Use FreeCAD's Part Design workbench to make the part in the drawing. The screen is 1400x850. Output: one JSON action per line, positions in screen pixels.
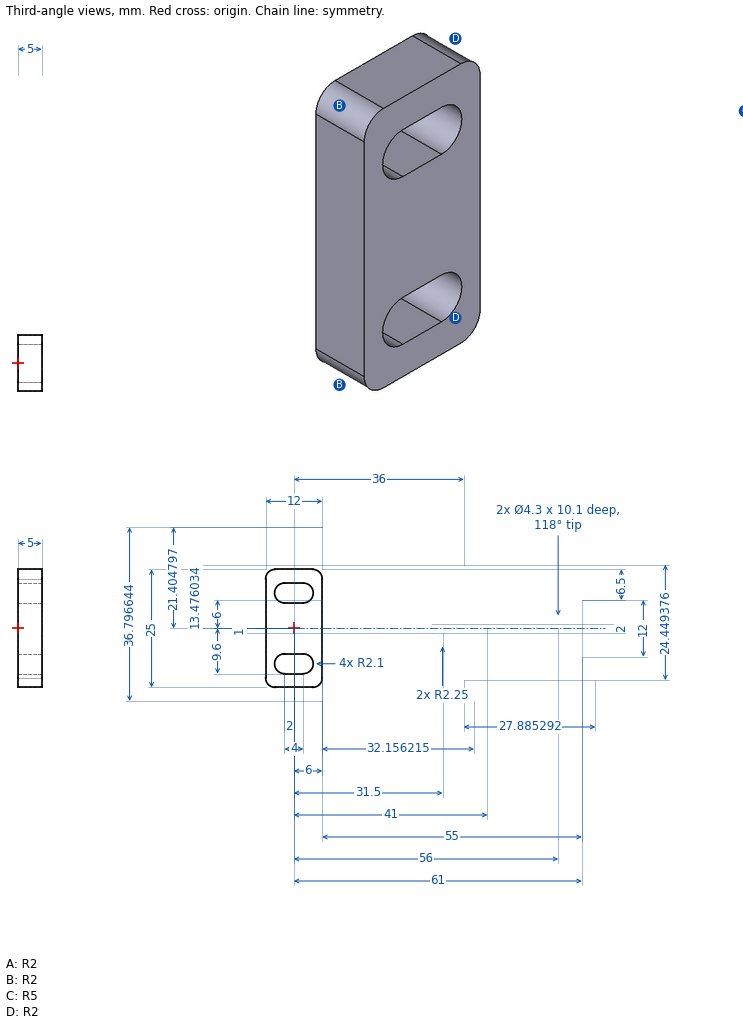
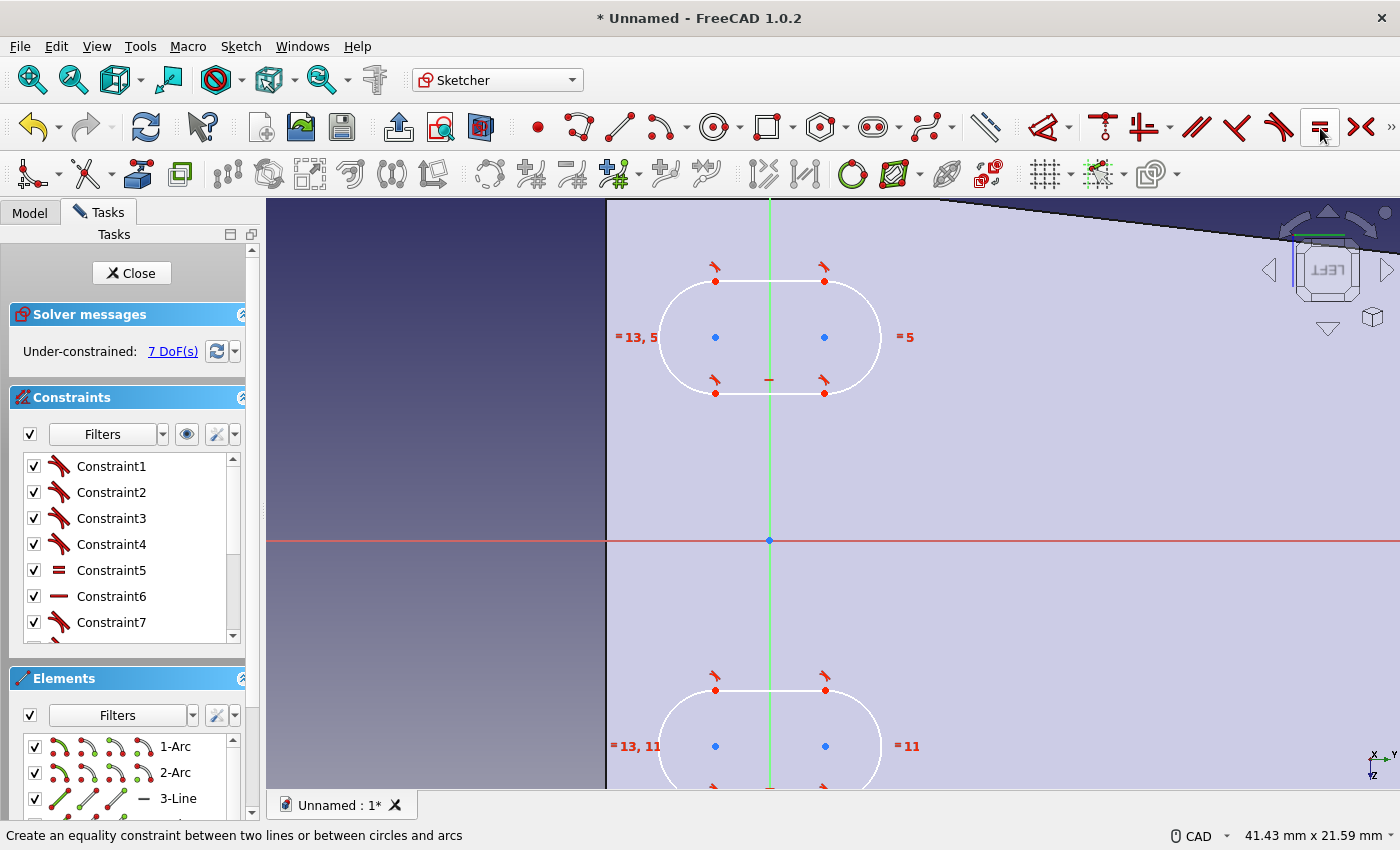
{"action": "left_click", "coordinate": [715, 338]}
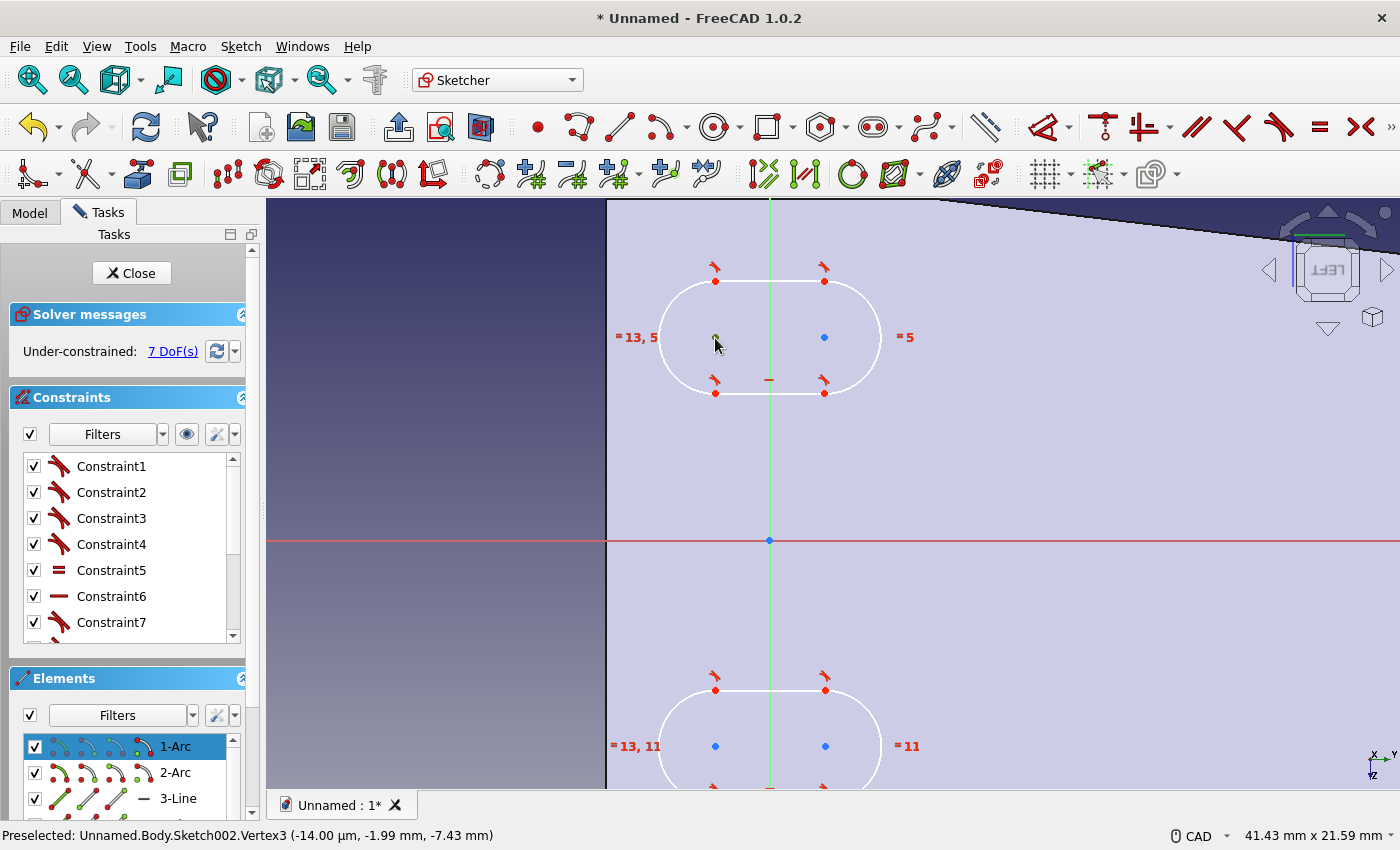
{"action": "left_click", "coordinate": [715, 747]}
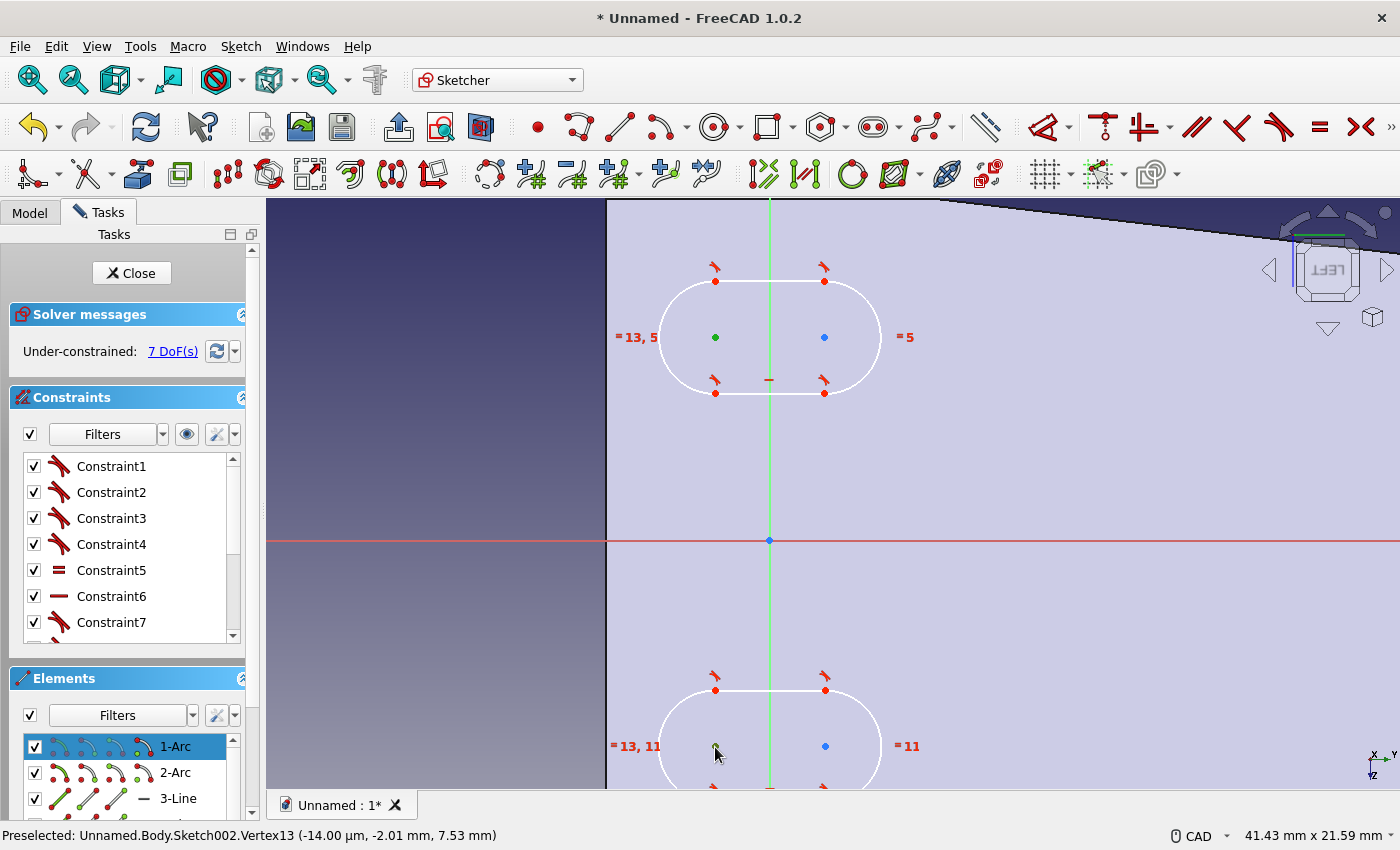
{"action": "left_click", "coordinate": [361, 541]}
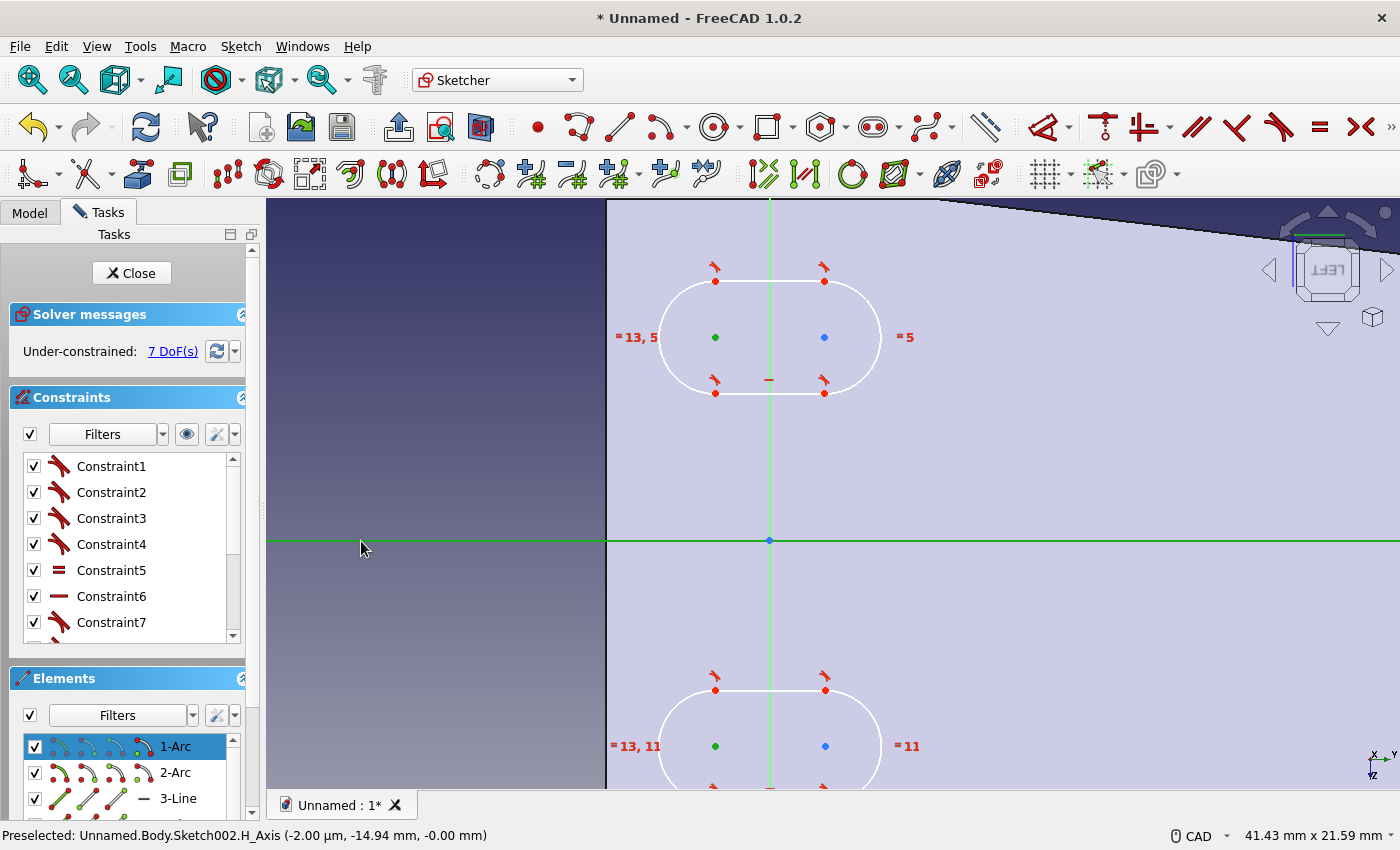
{"action": "left_click", "coordinate": [1361, 128]}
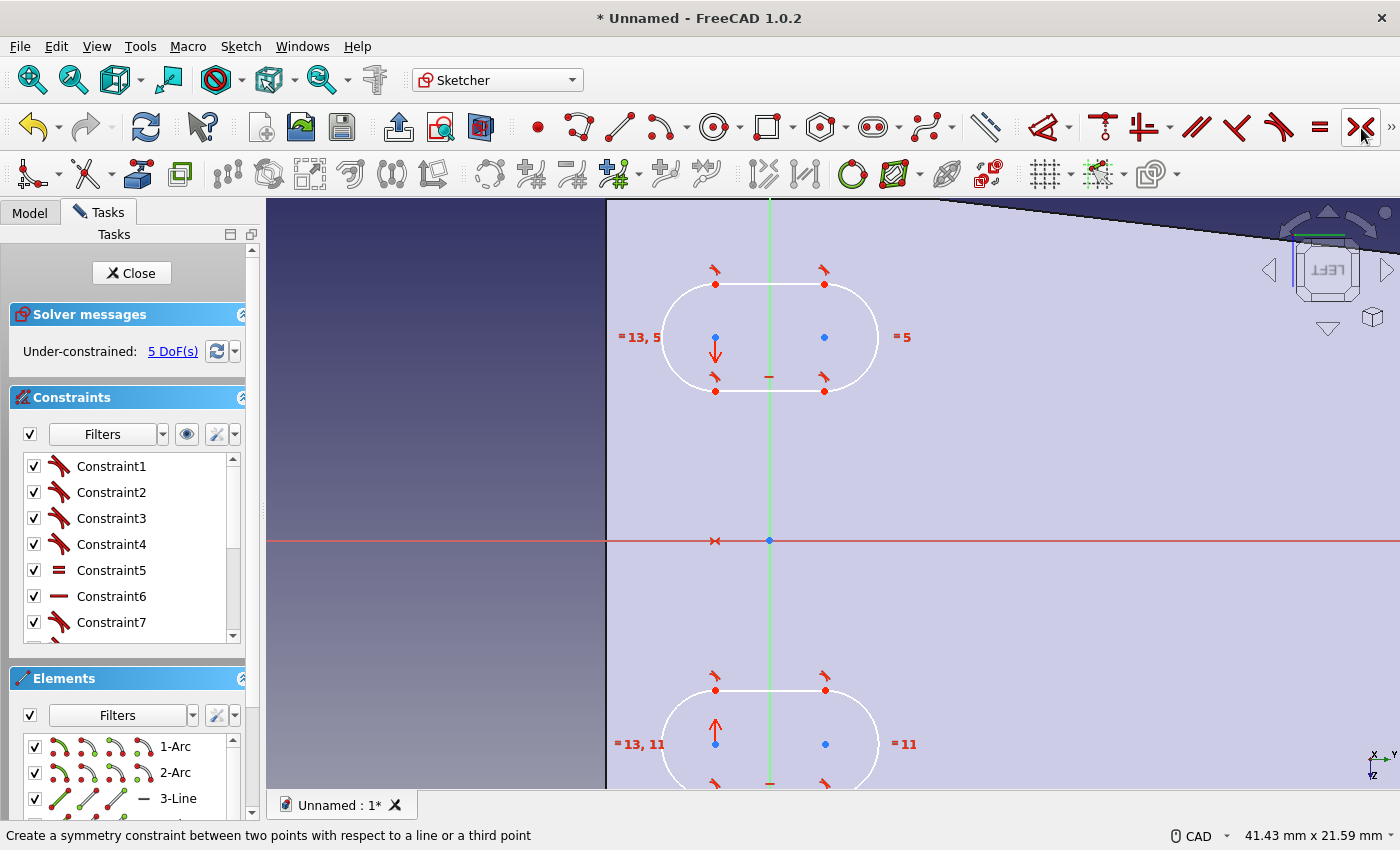
{"action": "left_click", "coordinate": [1042, 128]}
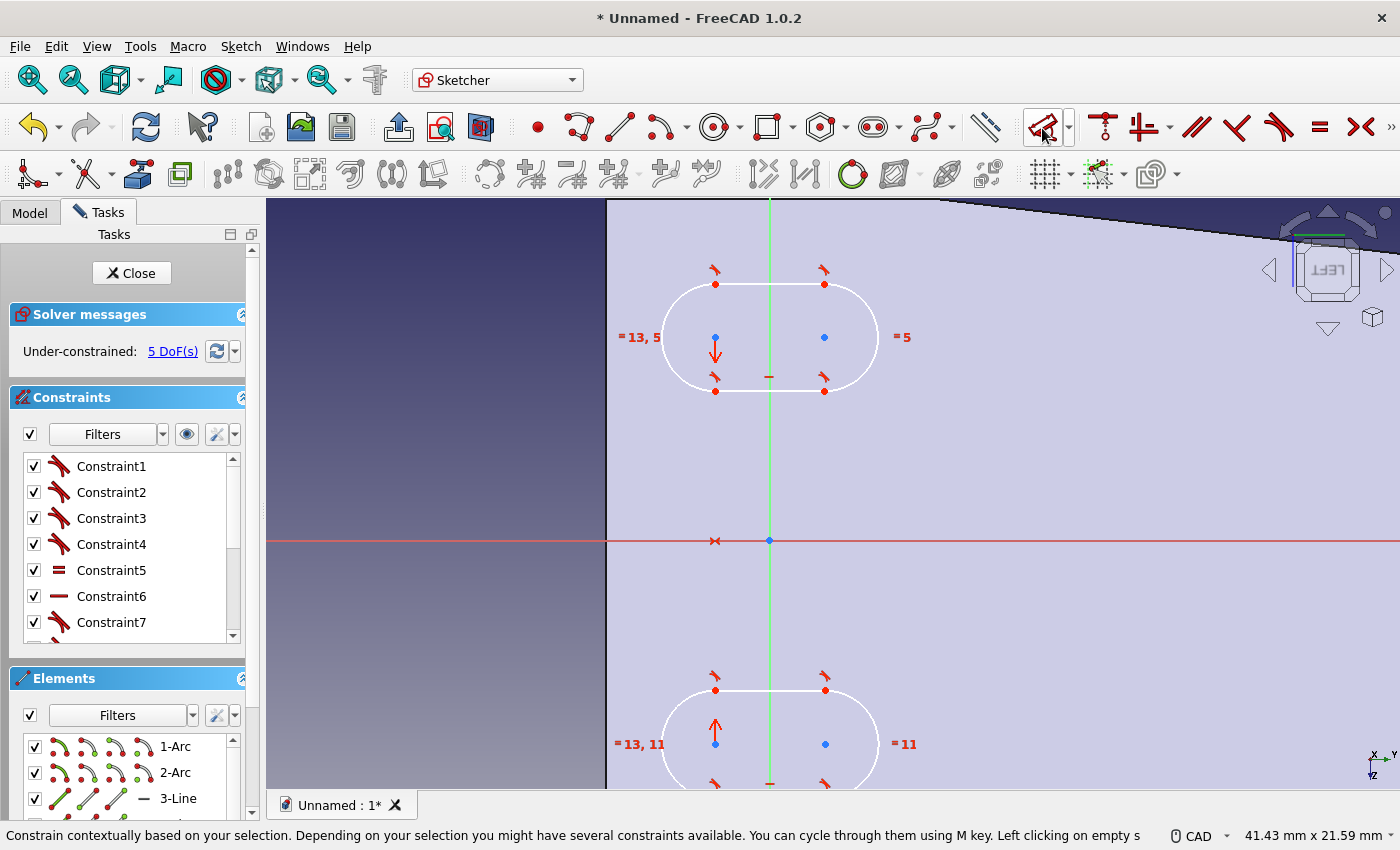
{"action": "left_click", "coordinate": [672, 306]}
{"action": "left_click", "coordinate": [646, 287]}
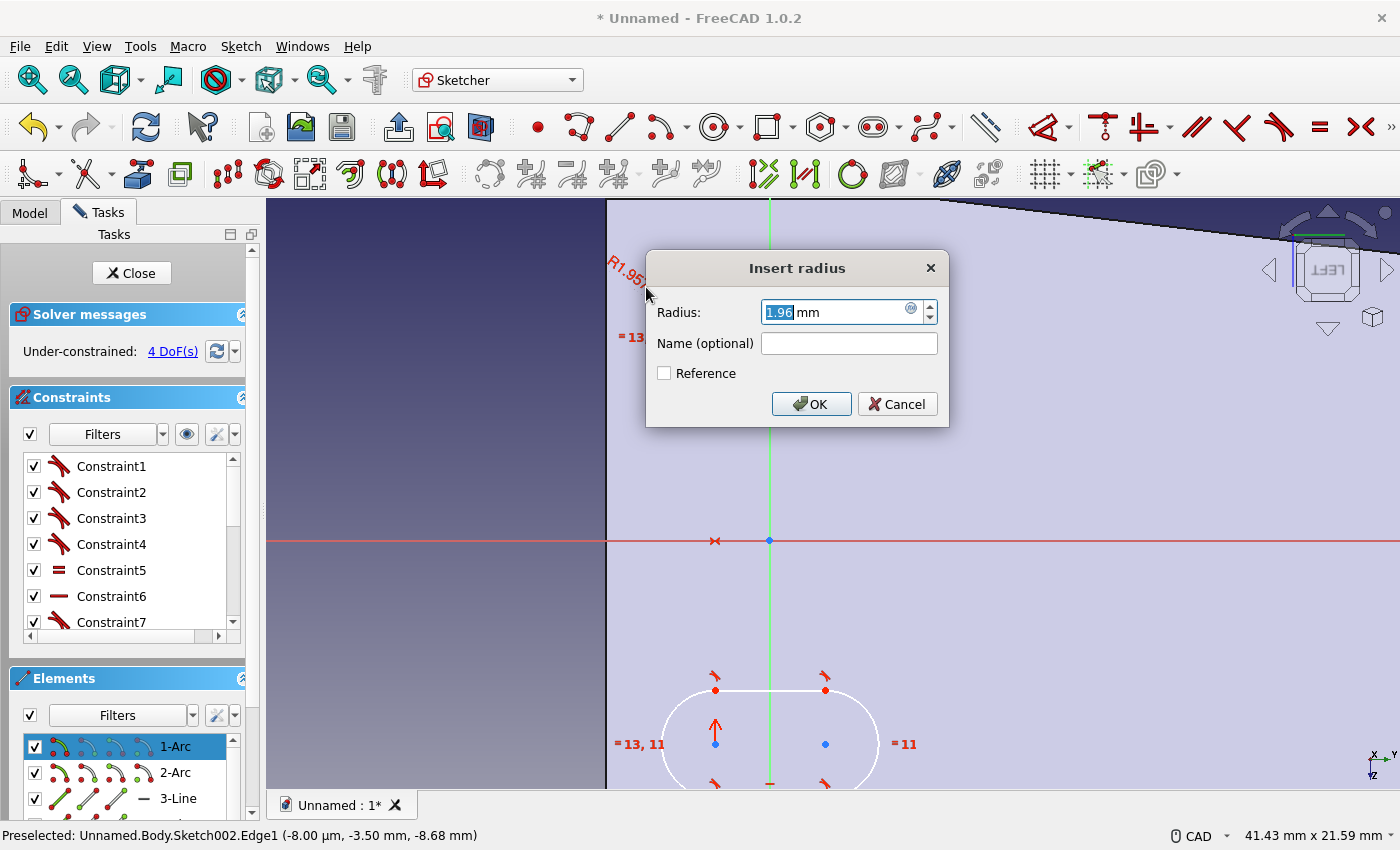
{"action": "type", "text": "2.1"}
{"action": "key", "text": "Return"}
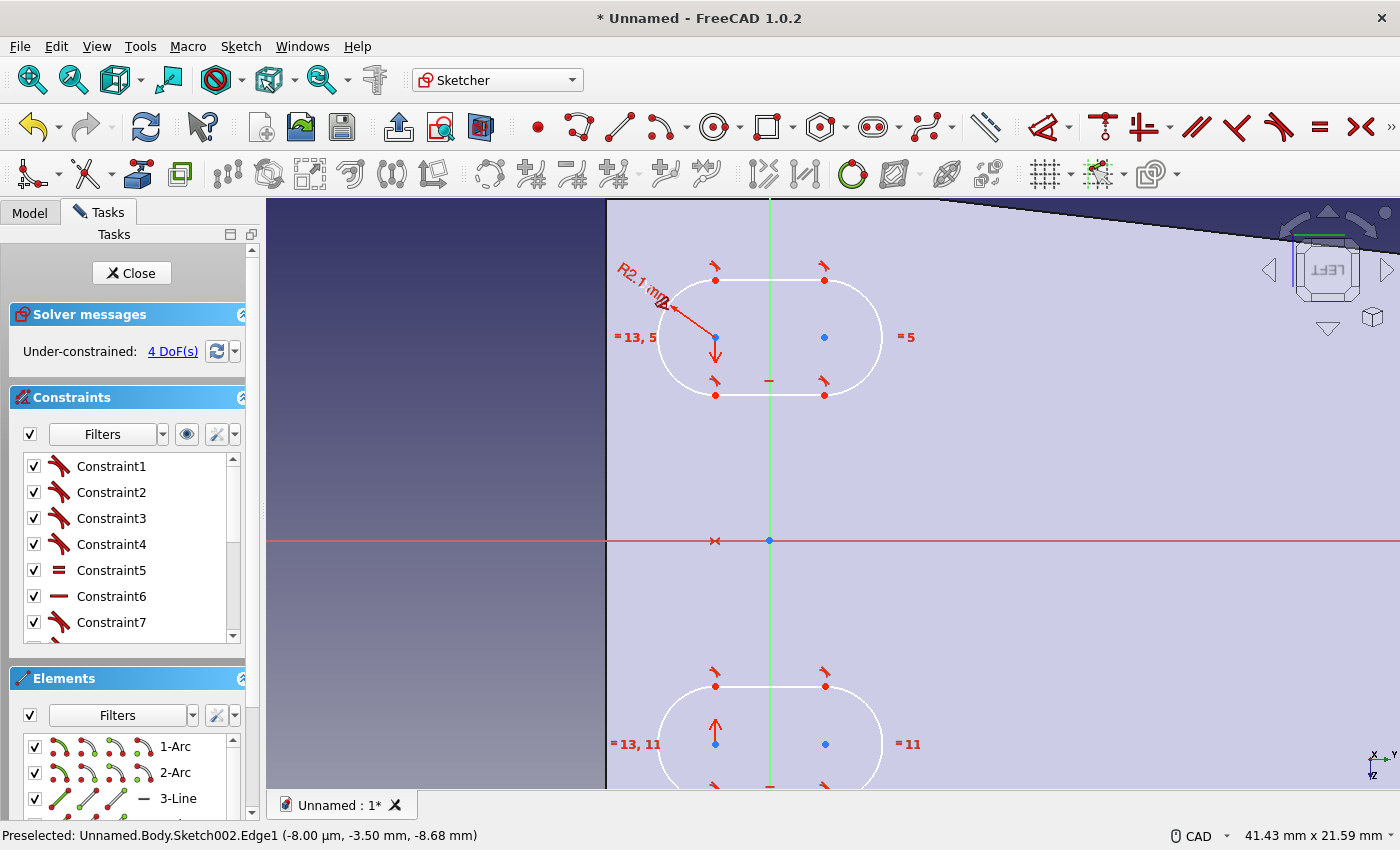
{"action": "left_click", "coordinate": [748, 280]}
{"action": "left_click", "coordinate": [745, 246]}